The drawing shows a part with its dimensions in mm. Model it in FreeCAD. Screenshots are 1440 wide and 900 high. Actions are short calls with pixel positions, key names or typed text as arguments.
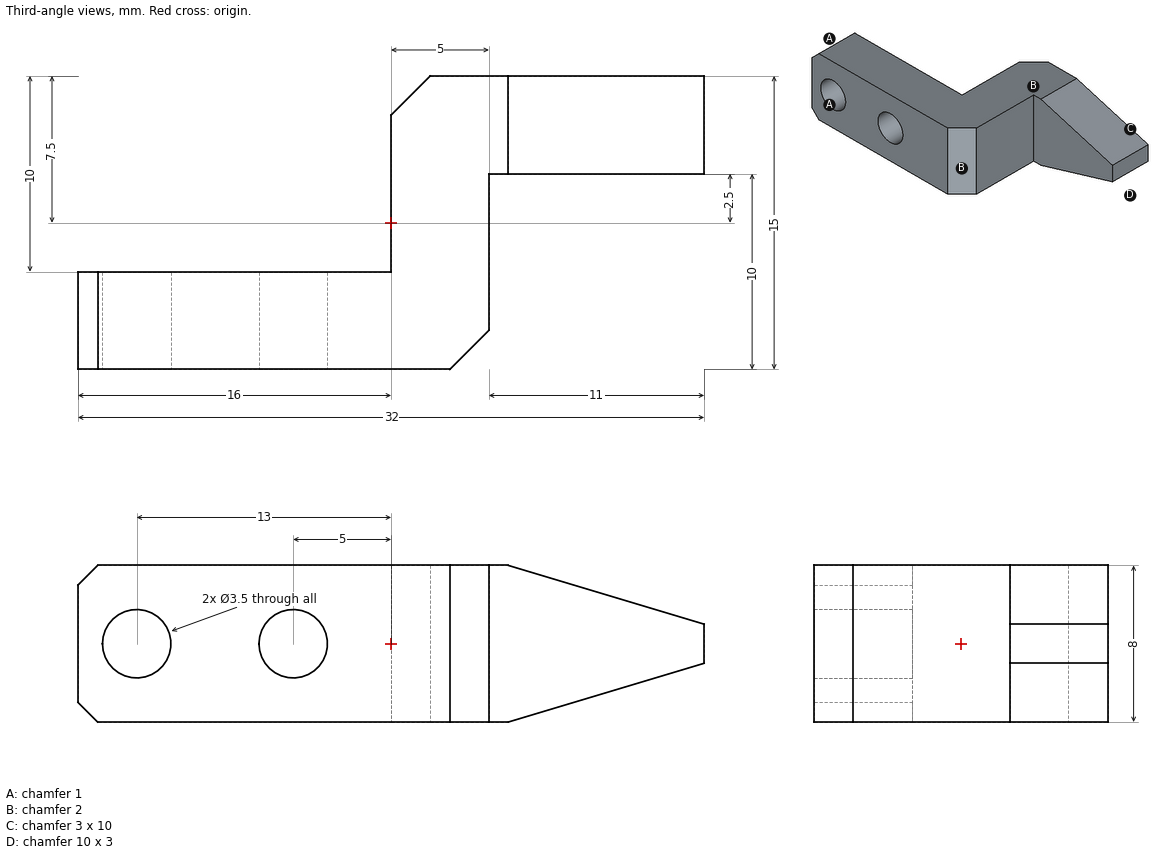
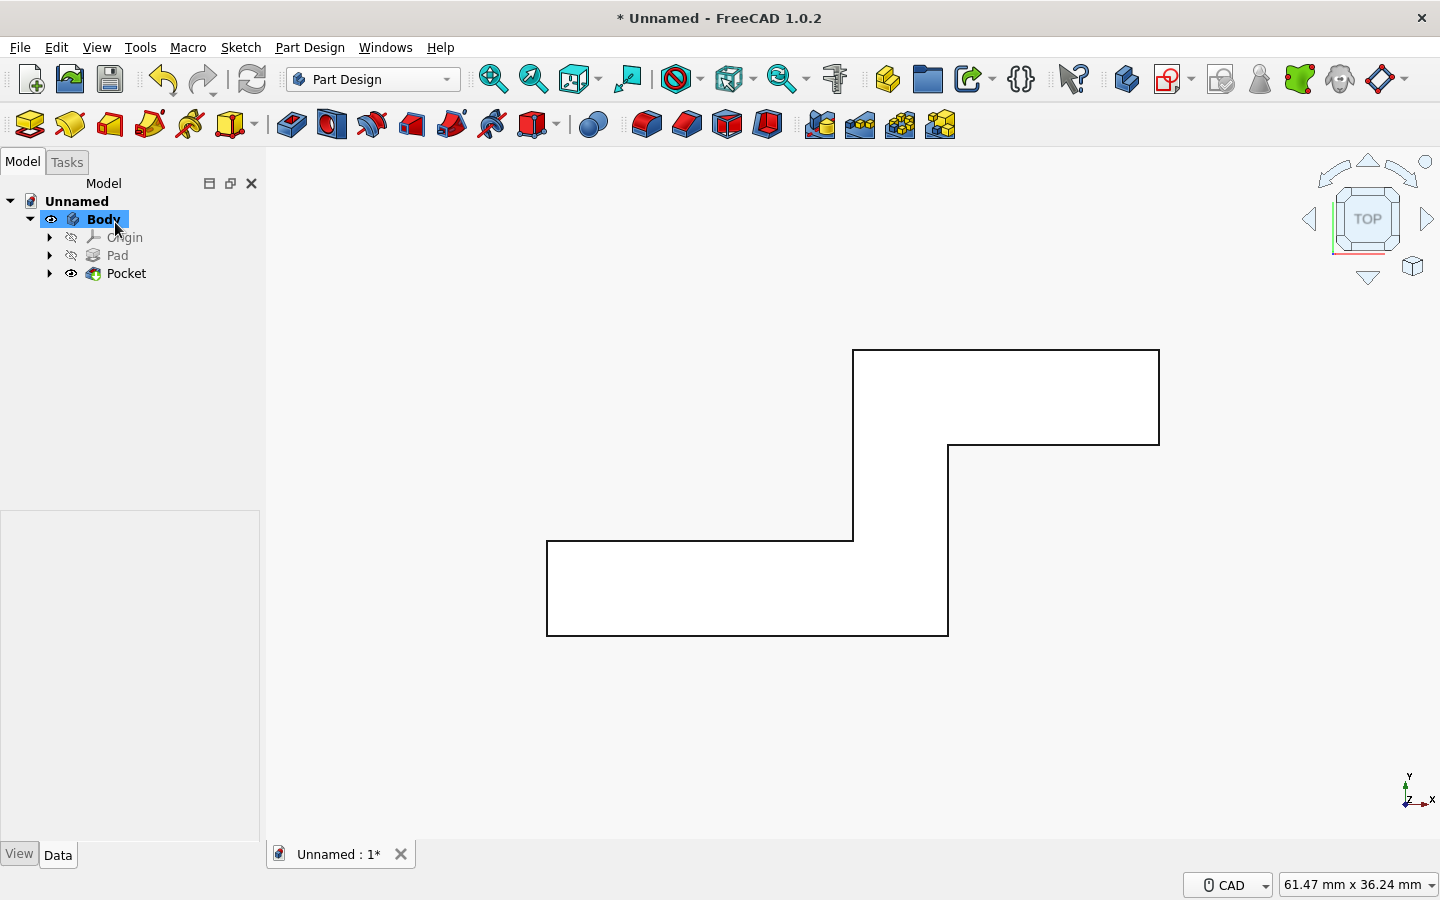
click(547, 587)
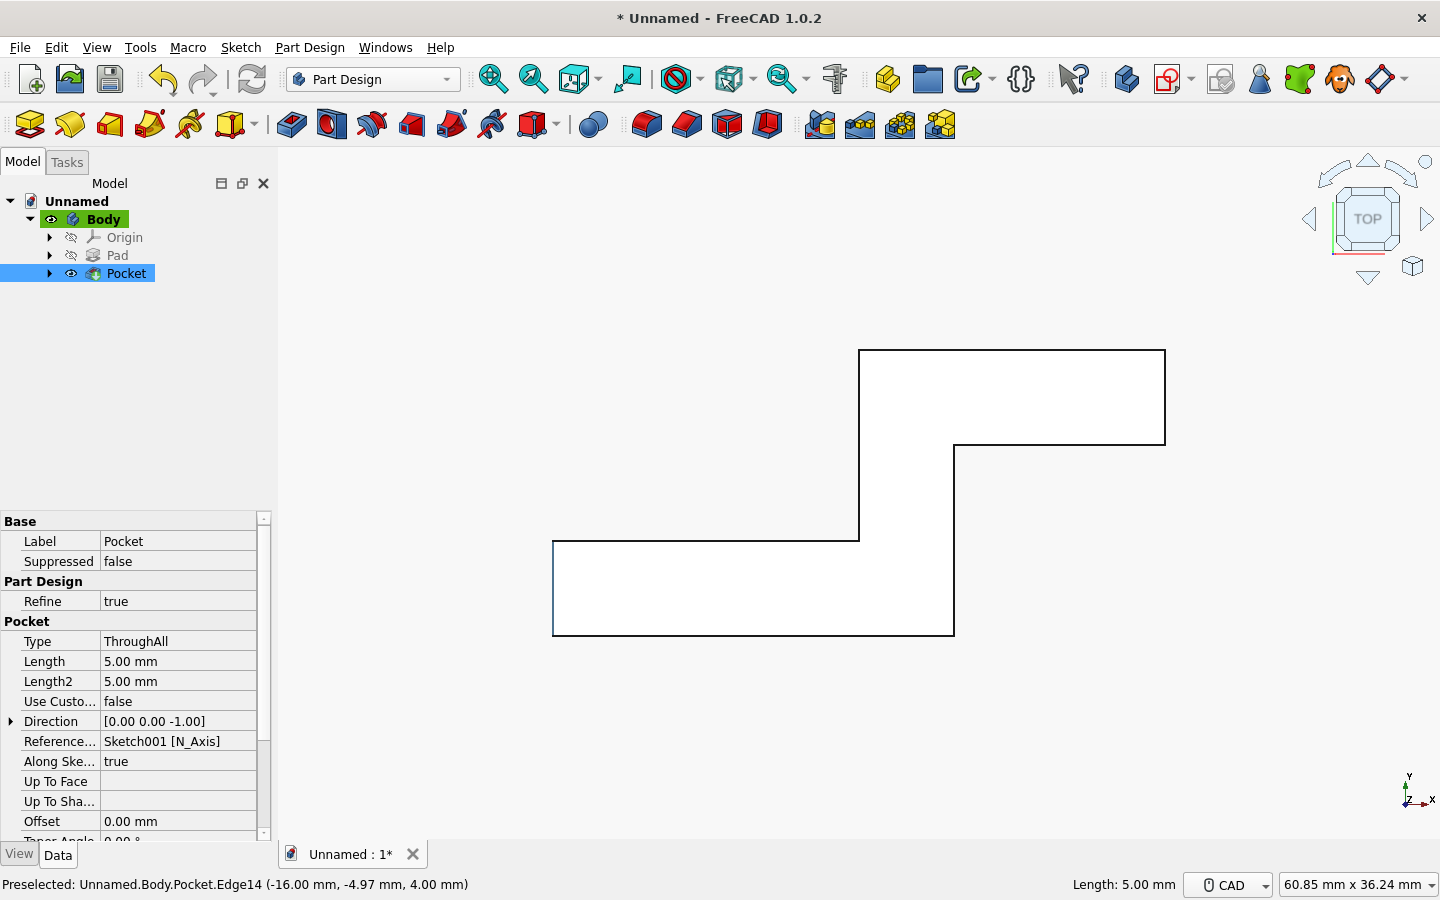
key(1)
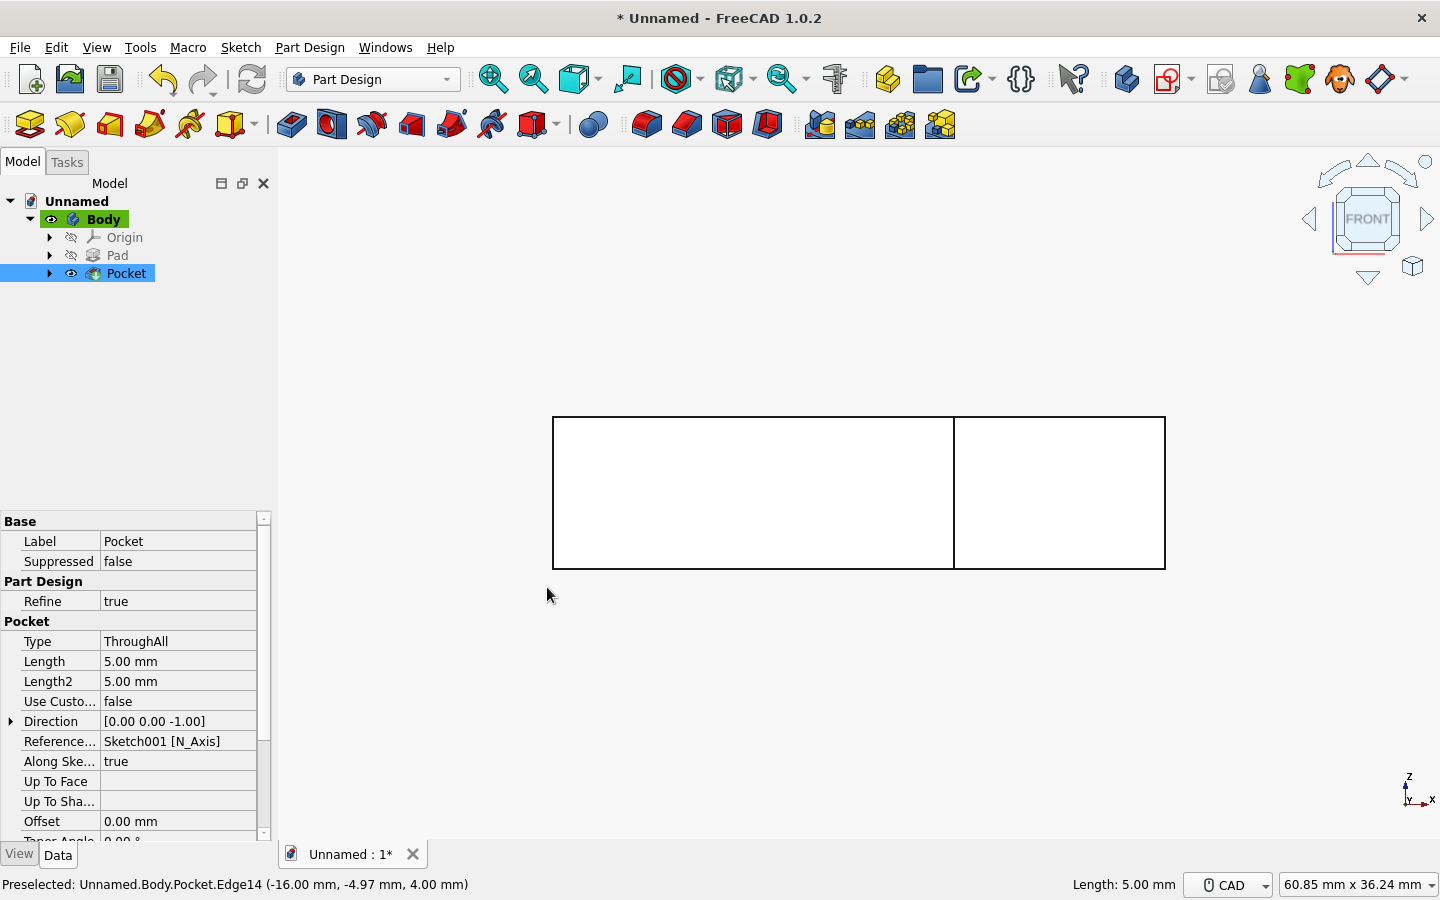
key(3)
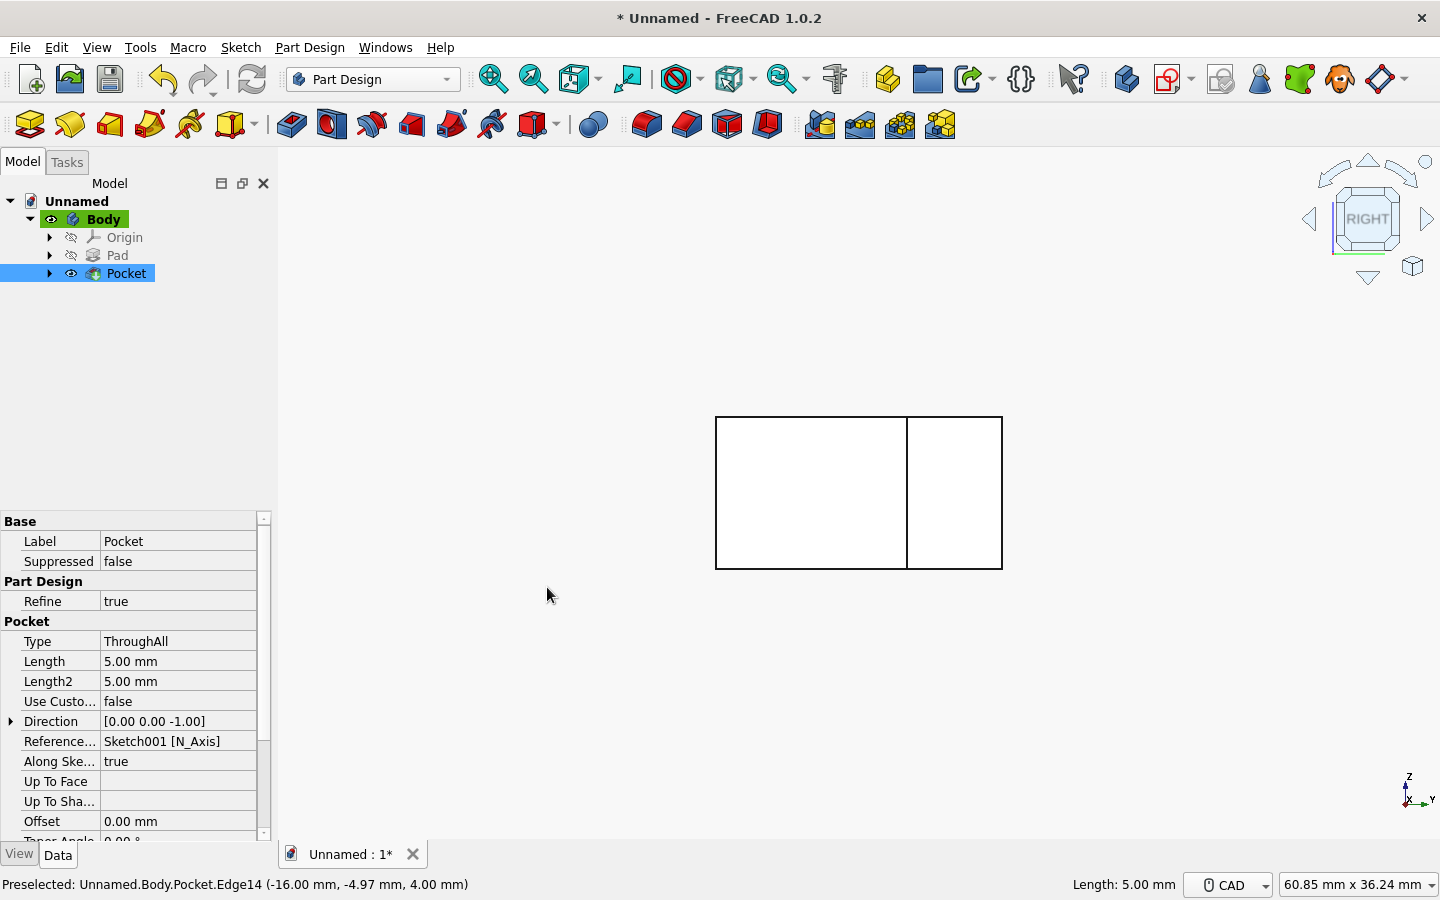
click(494, 80)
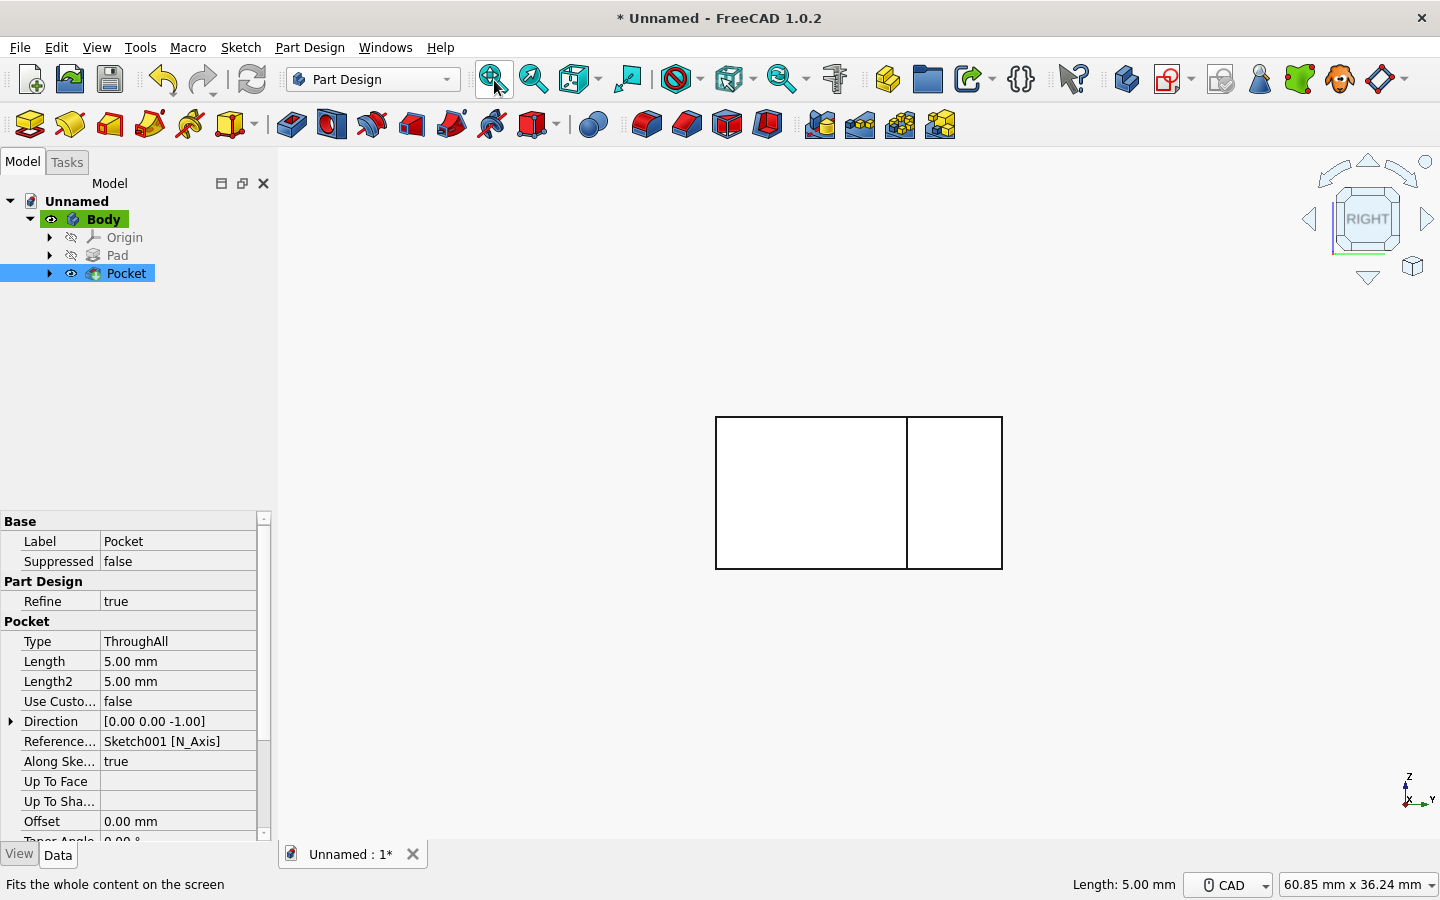
key(5)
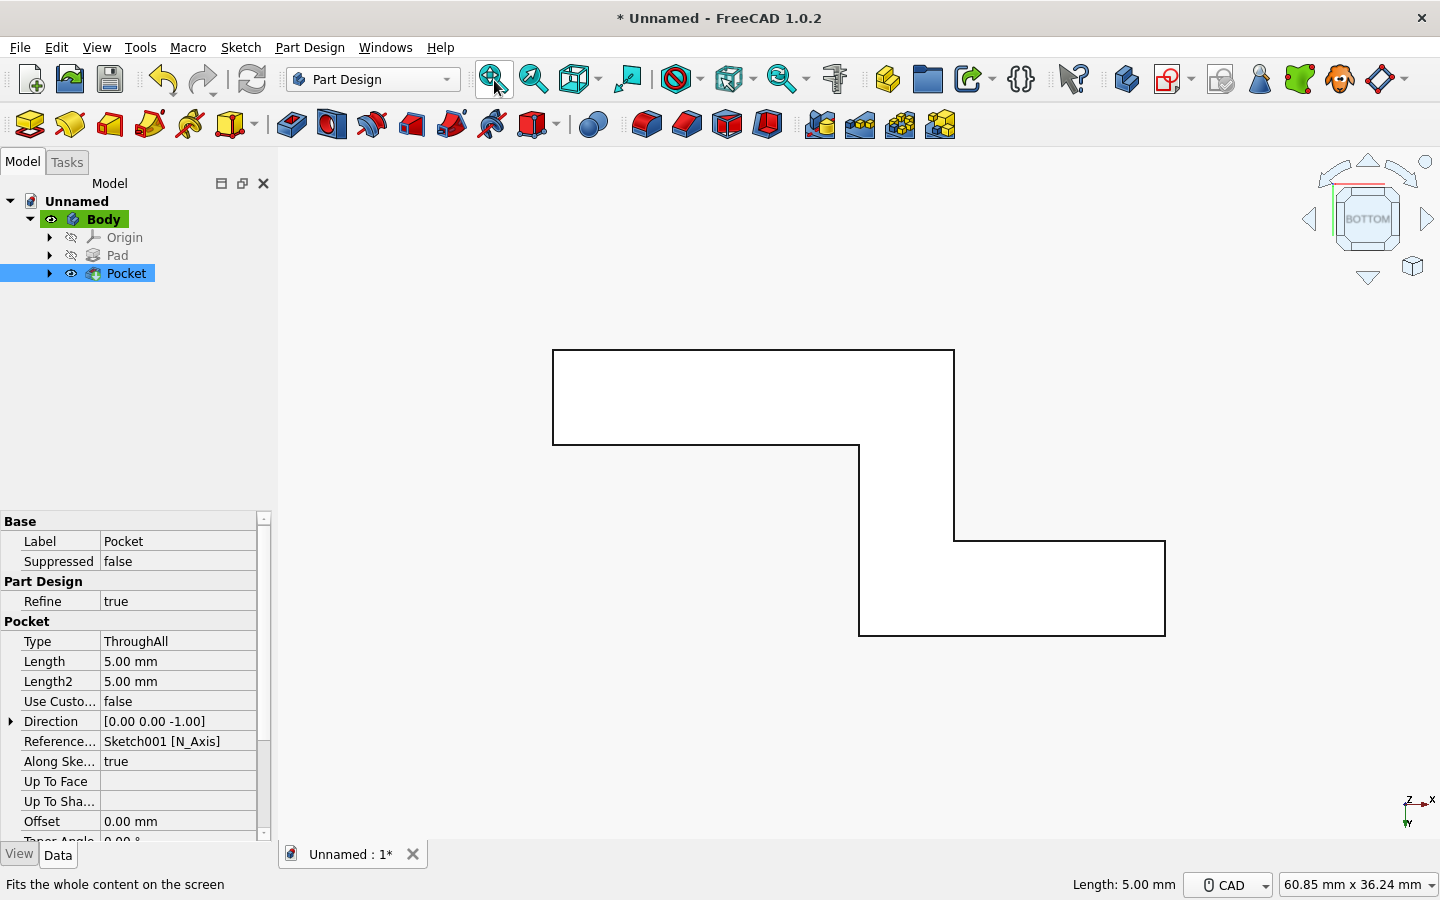
click(553, 397, ctrl)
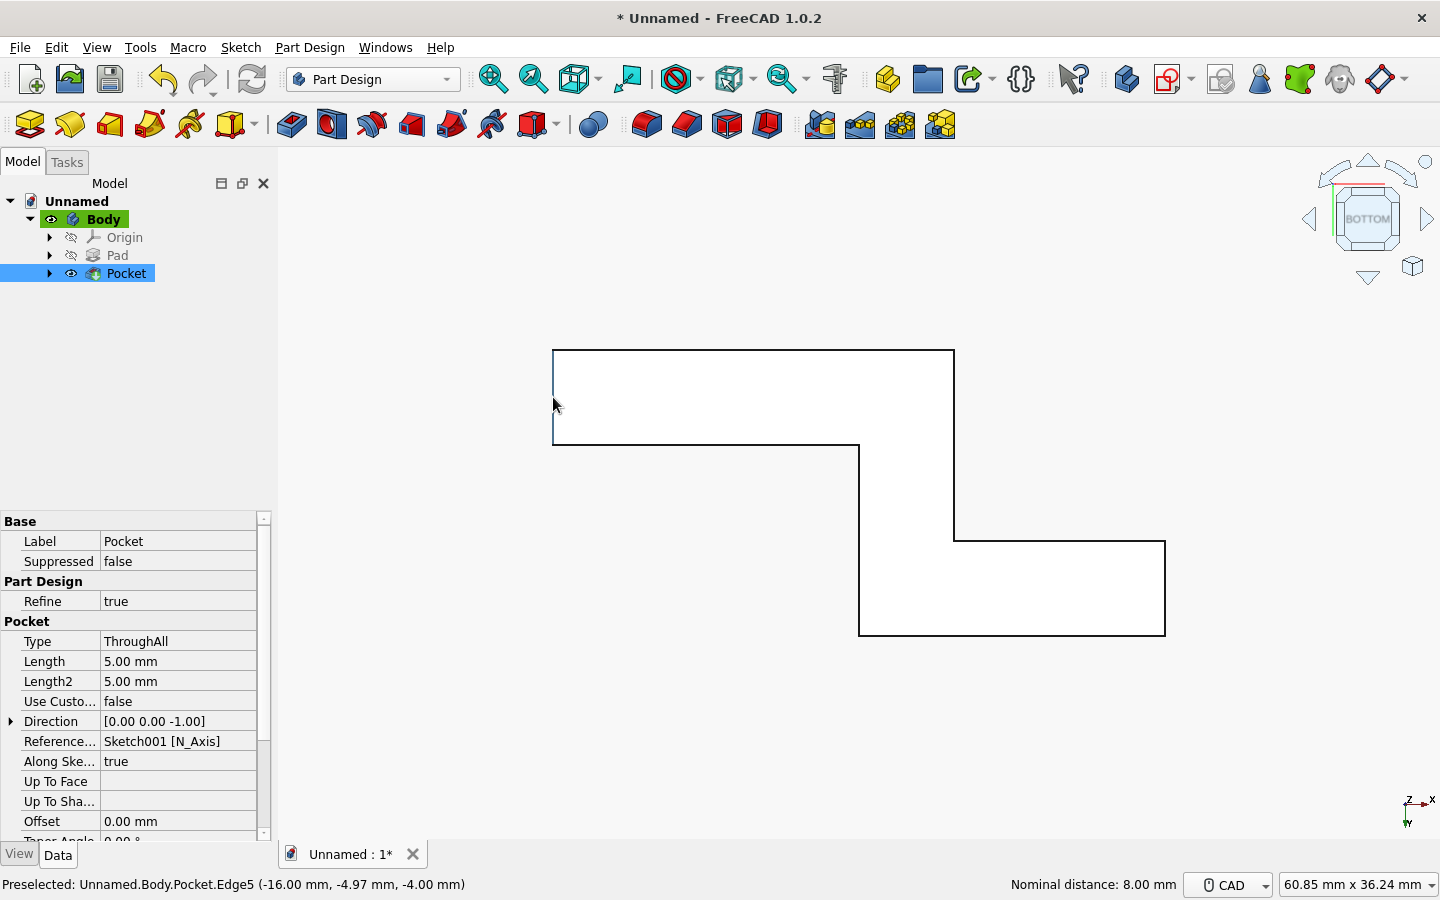
click(688, 124)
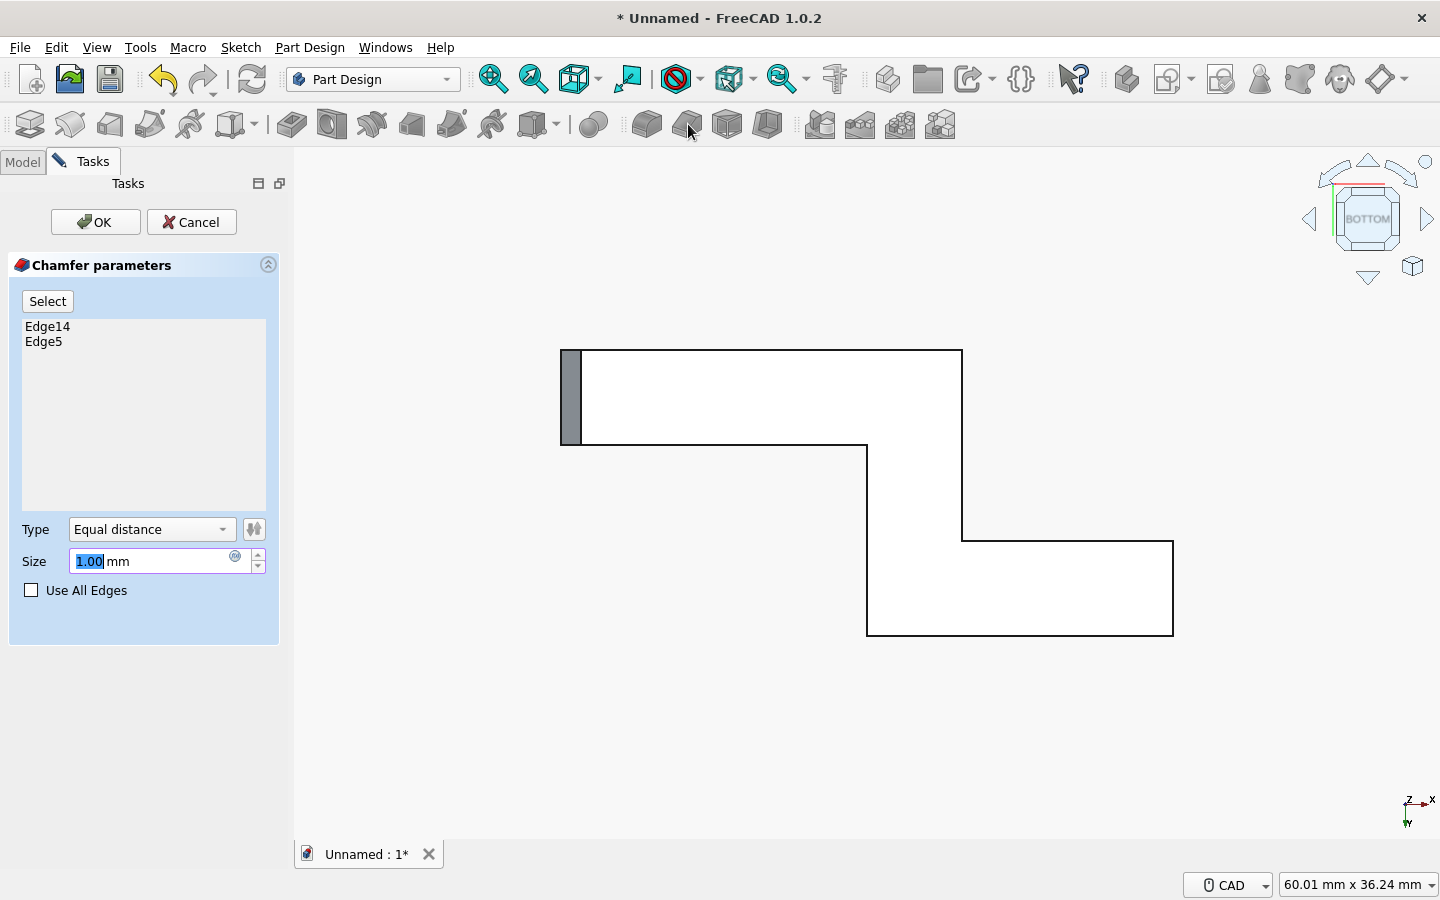
text(1)
key(Tab)